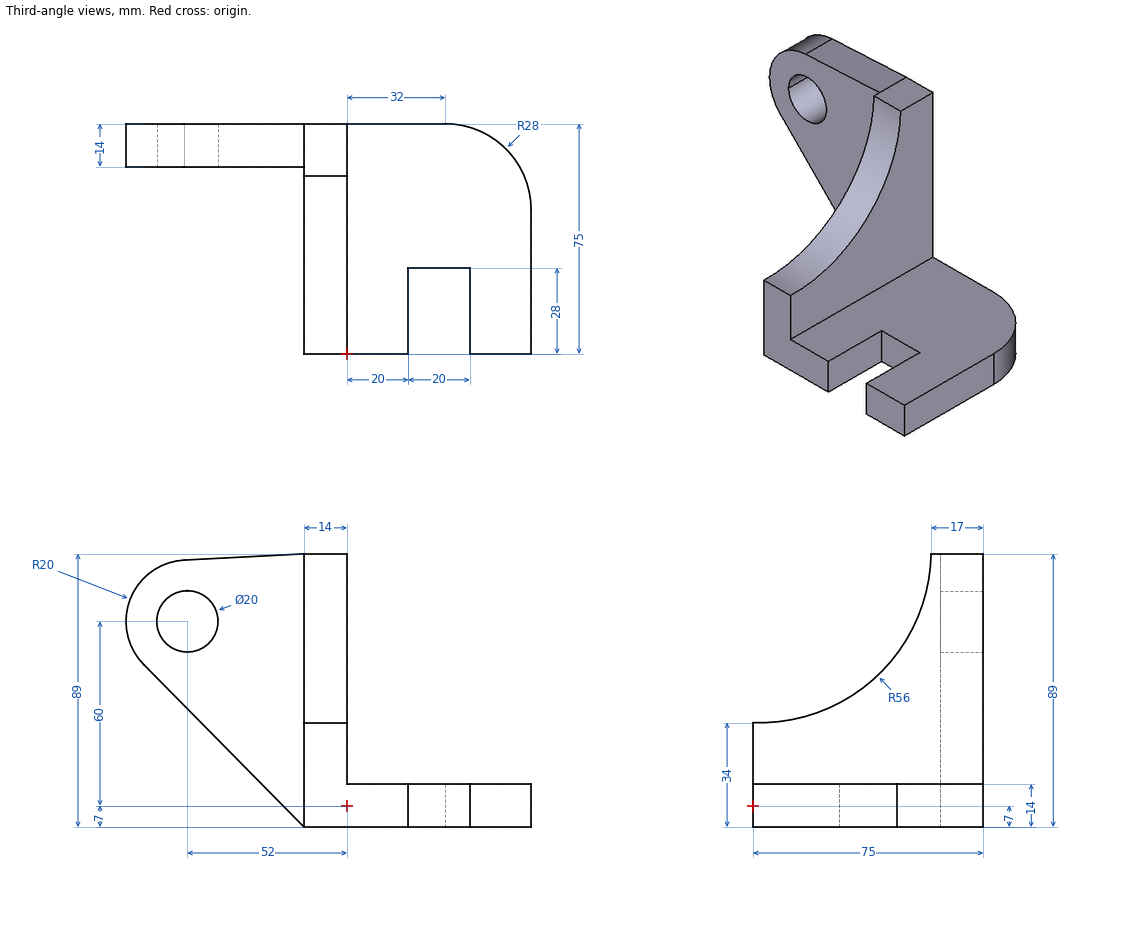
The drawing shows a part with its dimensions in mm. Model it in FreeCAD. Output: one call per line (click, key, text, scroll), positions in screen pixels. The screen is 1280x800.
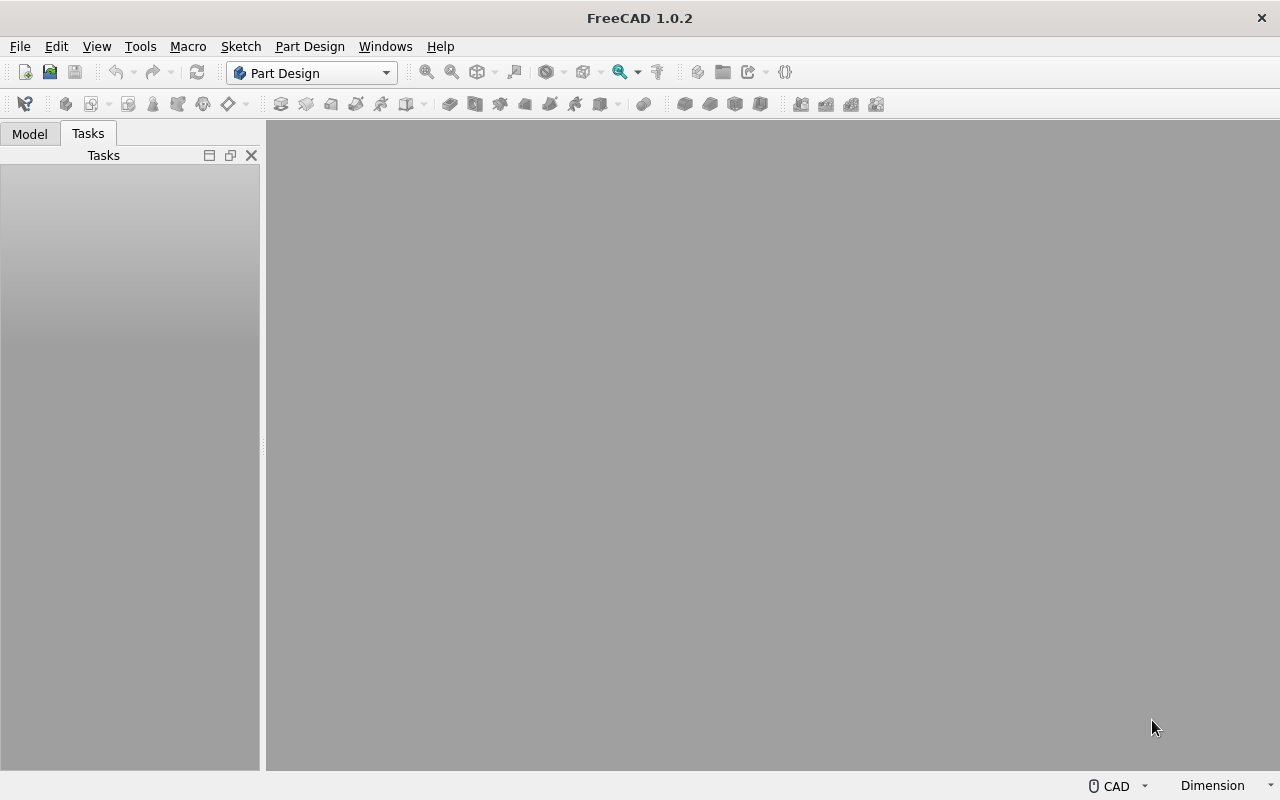
click(25, 72)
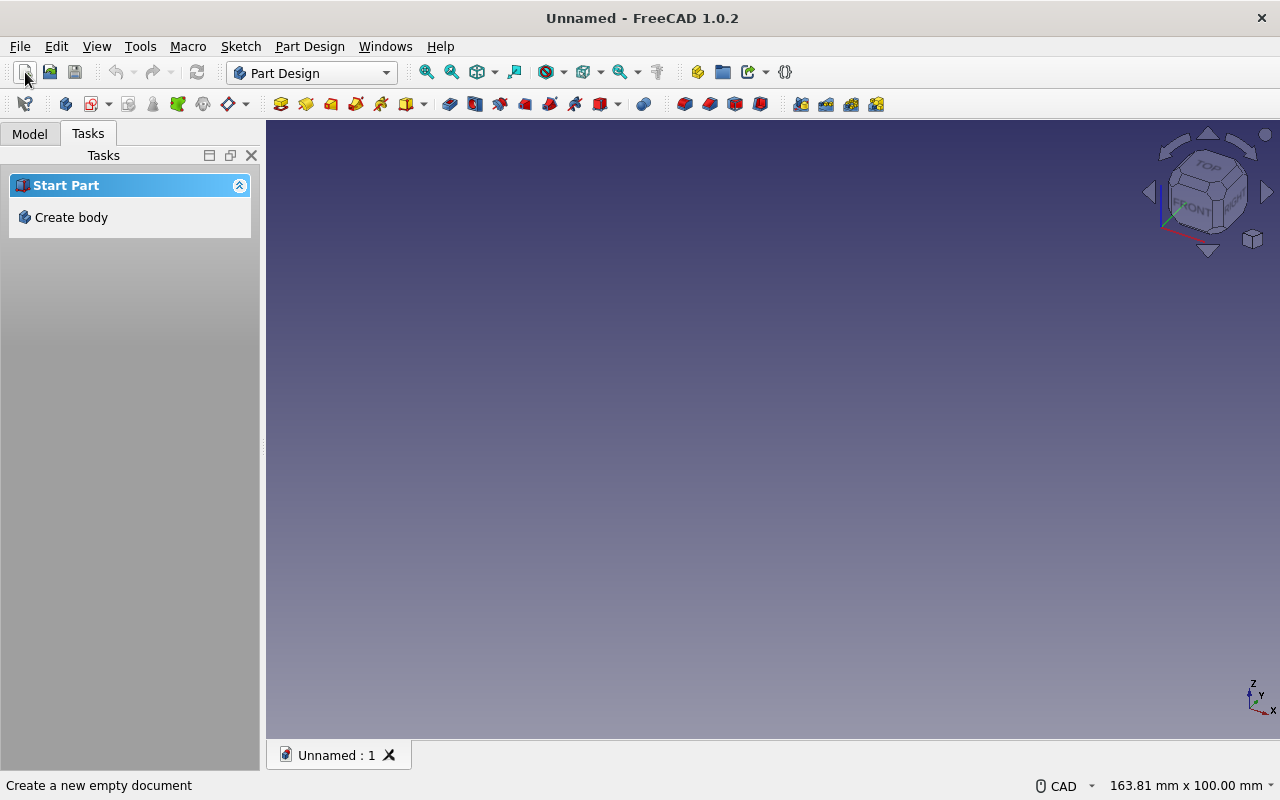
click(90, 104)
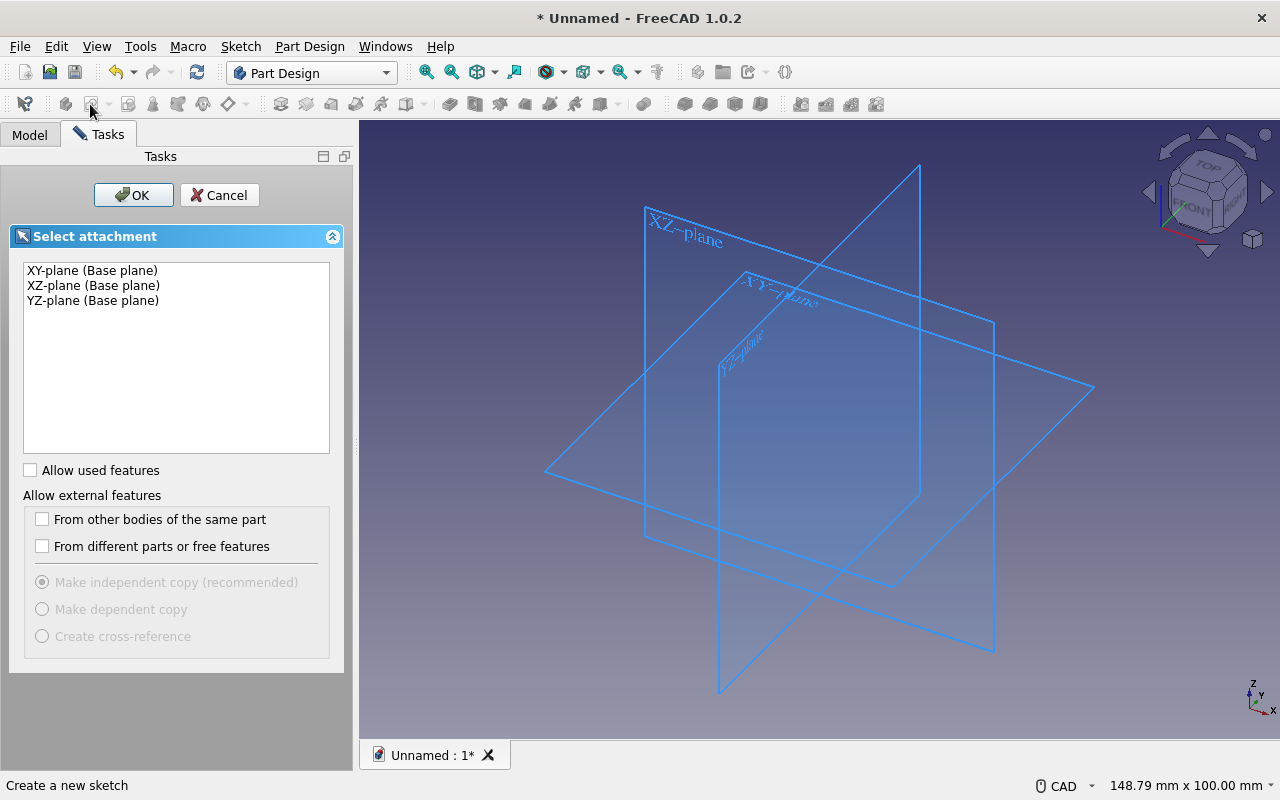
click(84, 270)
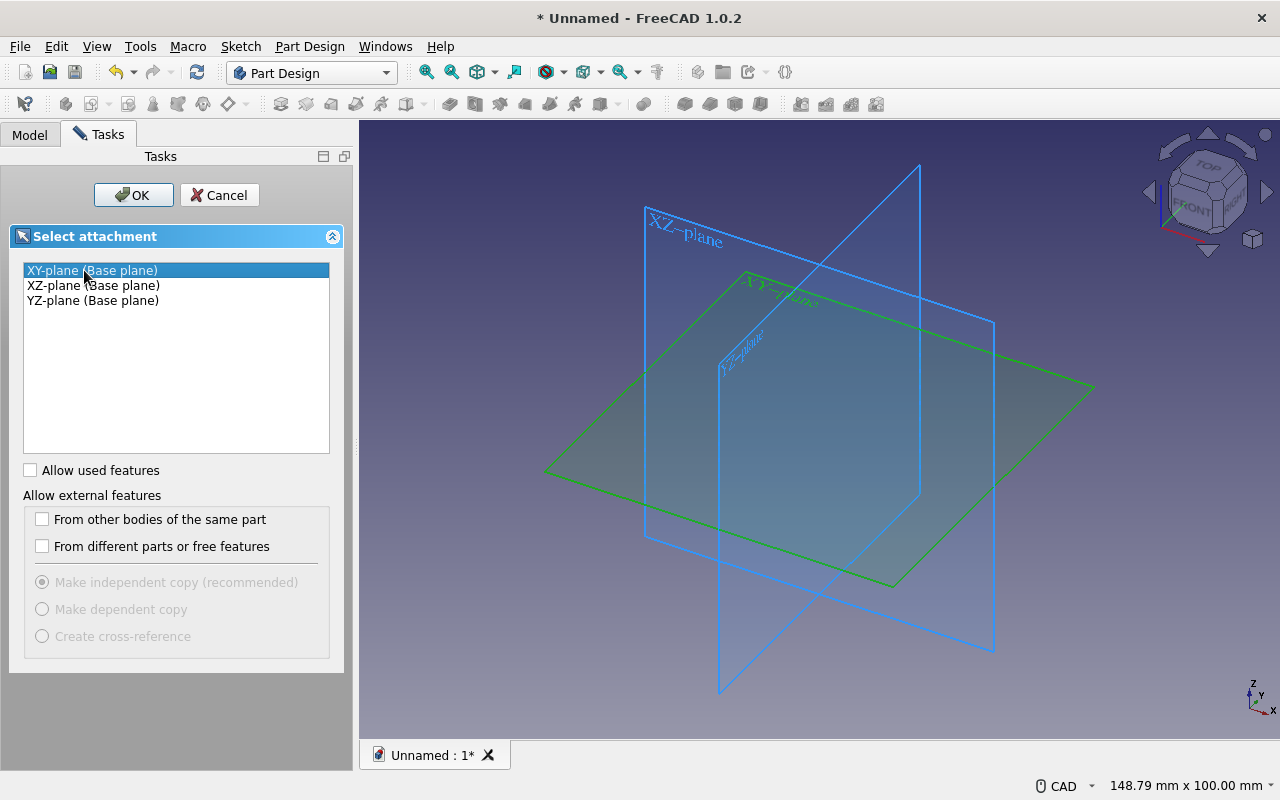
click(134, 195)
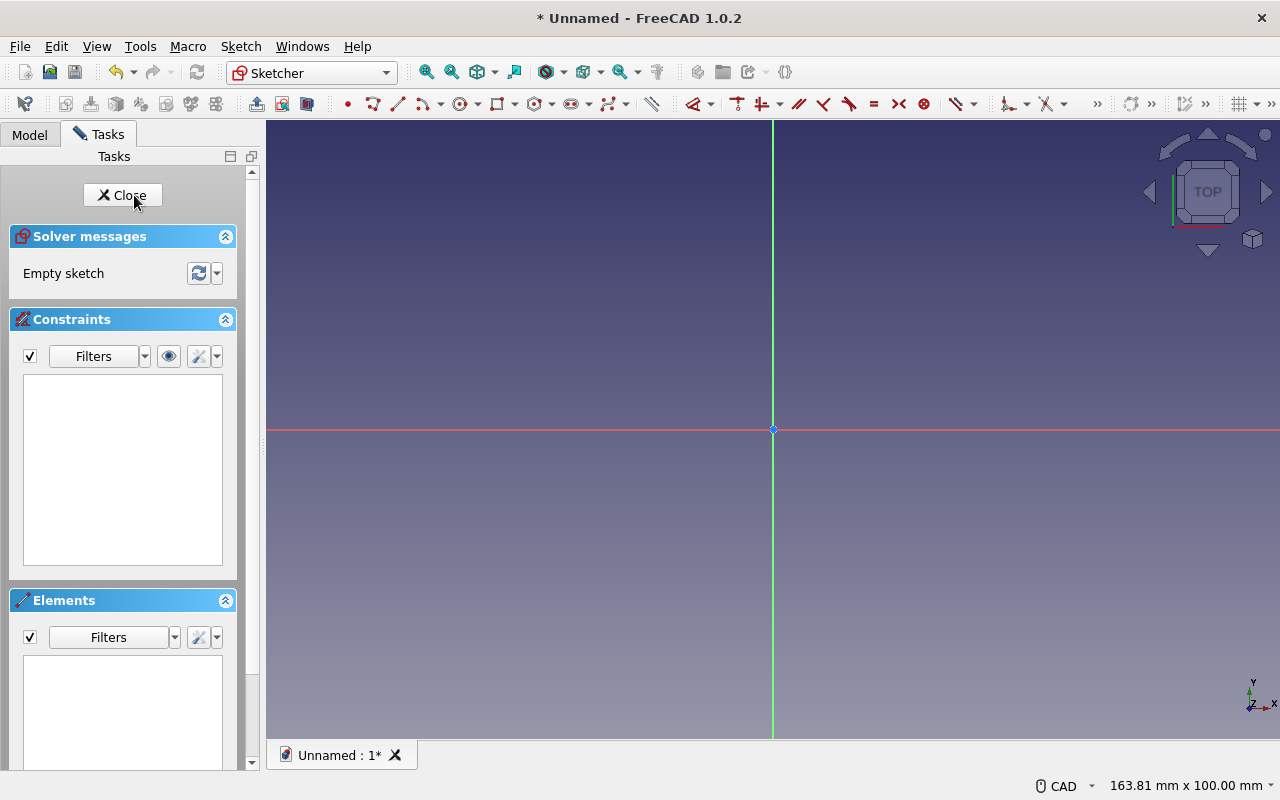
scroll(294, 711, down, 2)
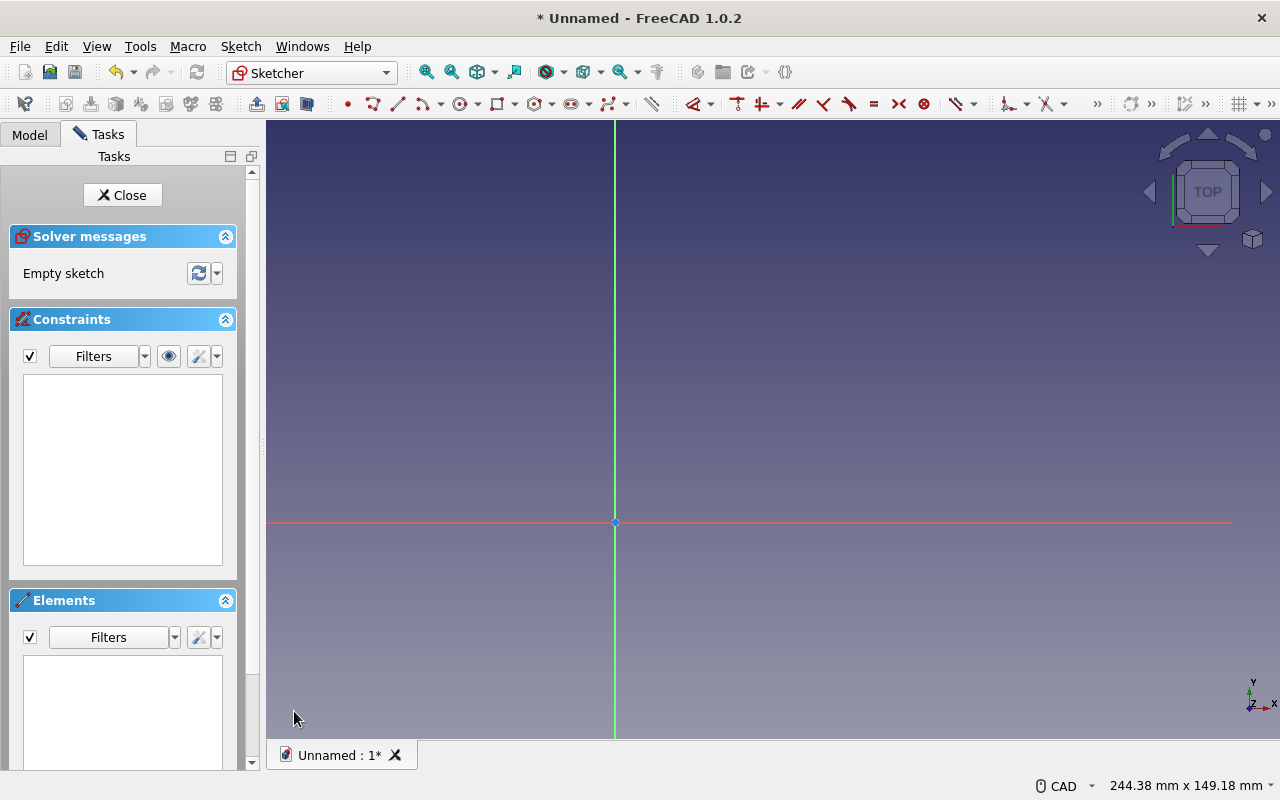
click(373, 104)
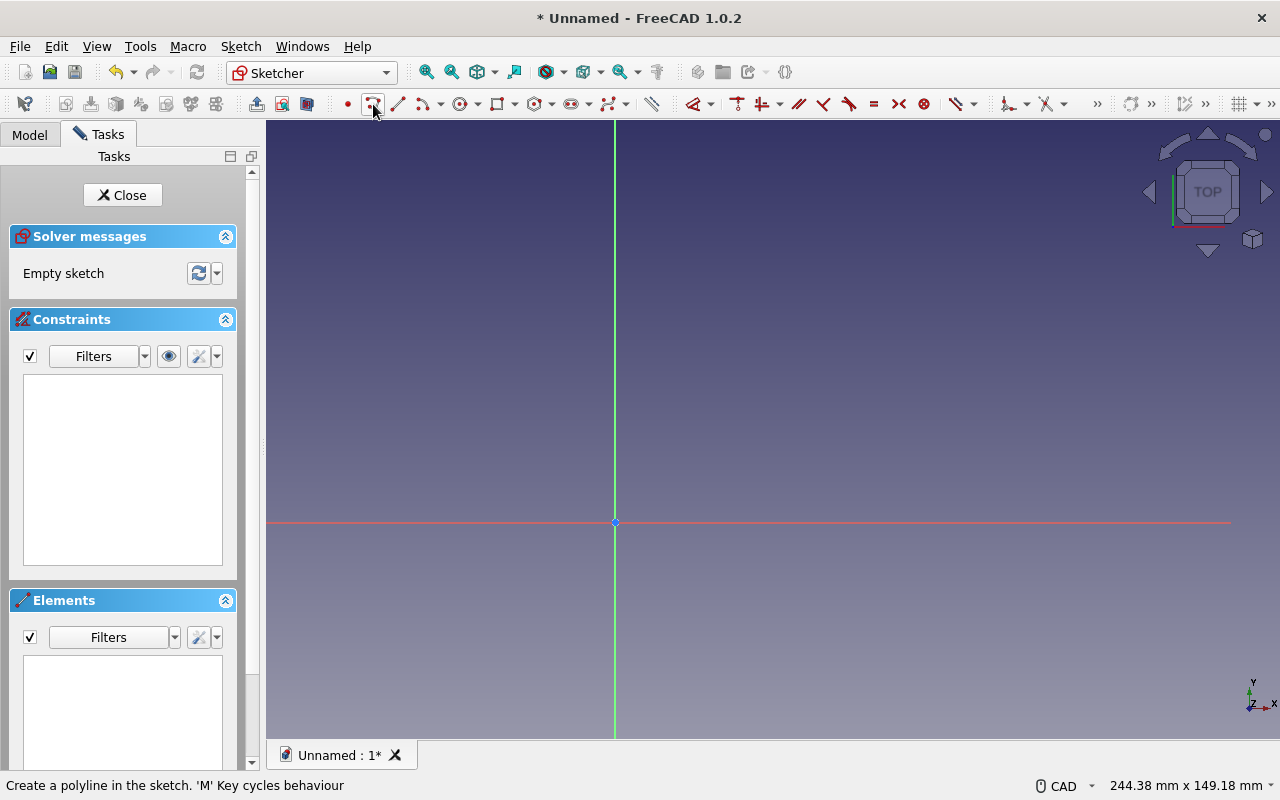
click(748, 211)
click(615, 211)
click(615, 523)
click(698, 514)
click(698, 406)
click(781, 406)
click(781, 523)
click(864, 514)
click(864, 328)
right_click(864, 328)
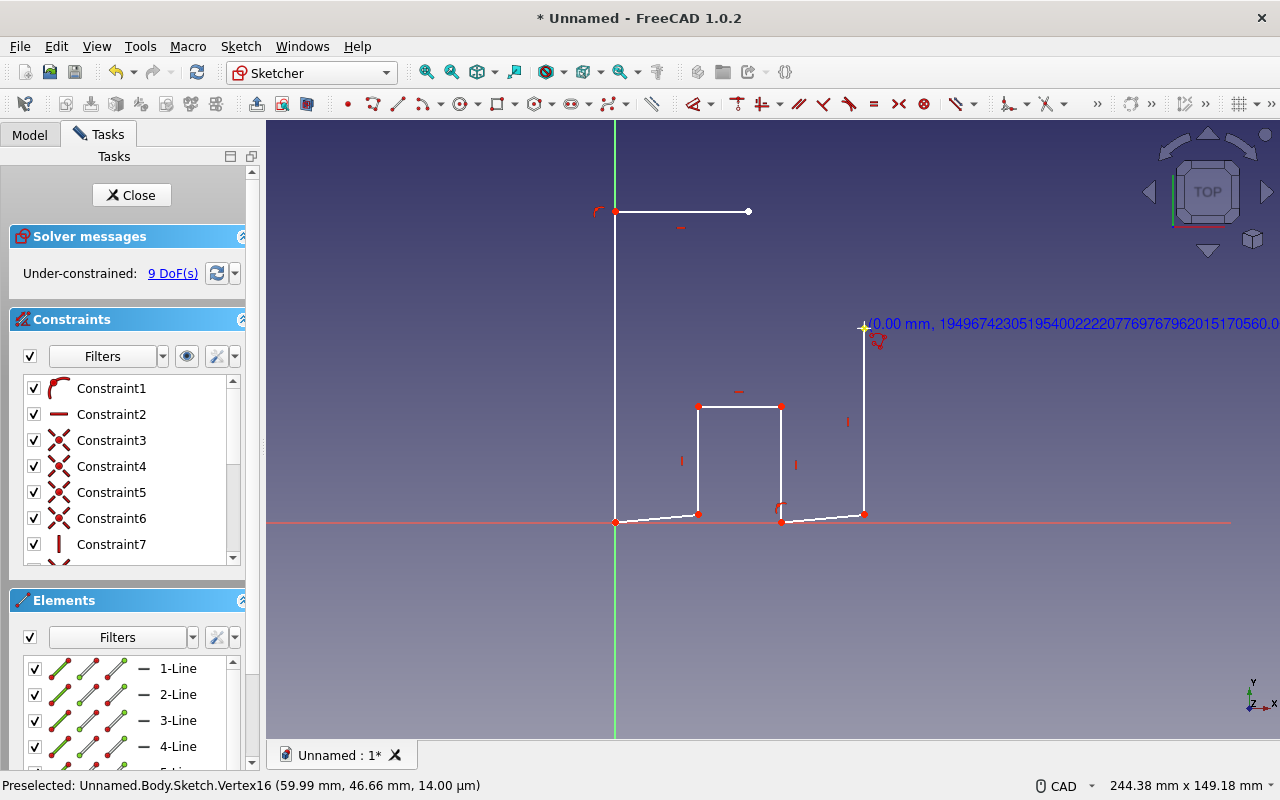
key(g)
key(3)
key(a)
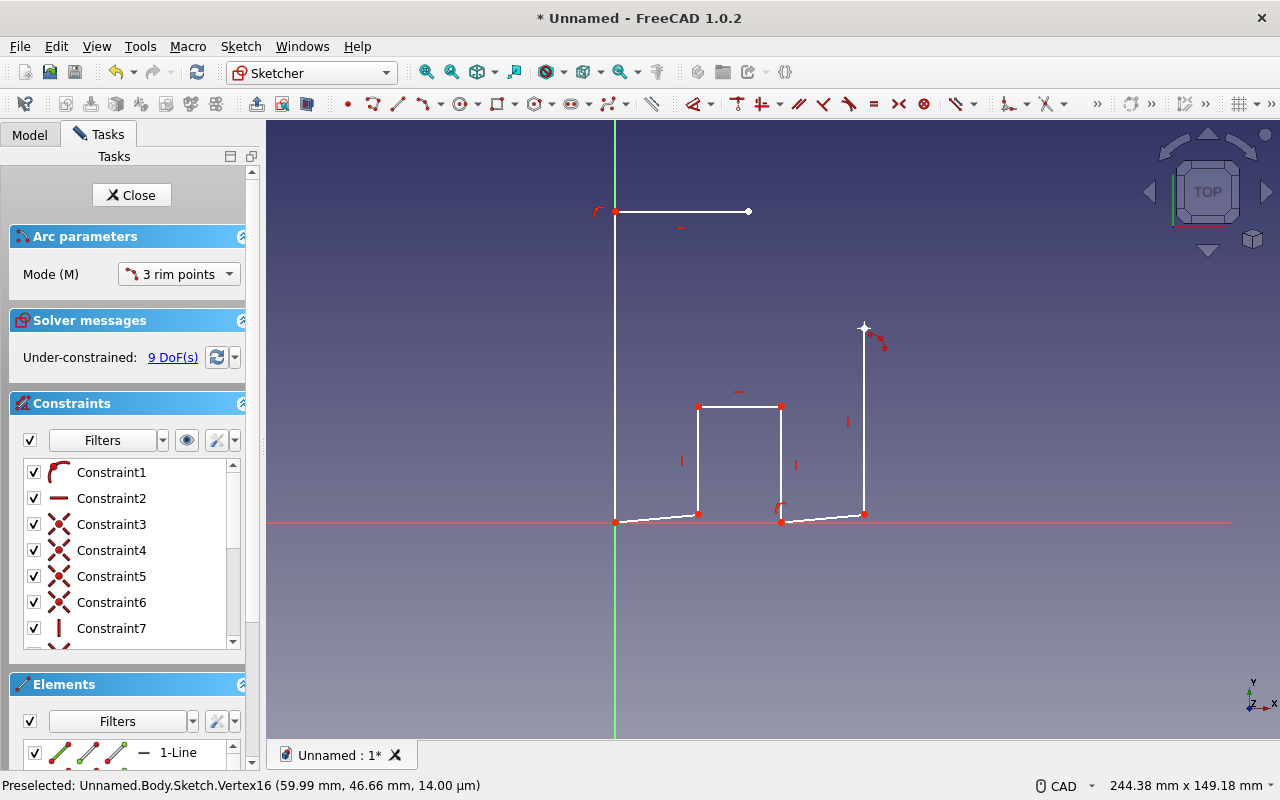
click(864, 329)
click(748, 212)
click(830, 245)
key(Escape)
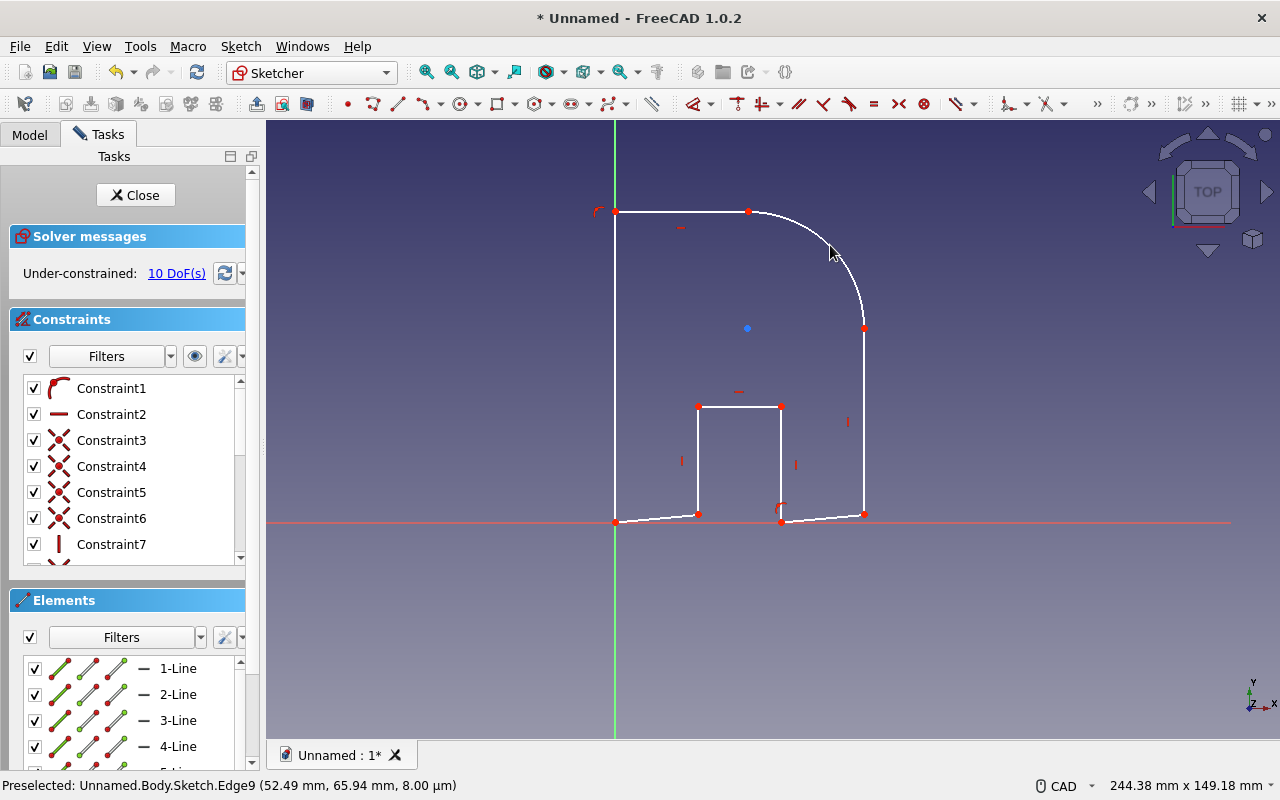
click(708, 212)